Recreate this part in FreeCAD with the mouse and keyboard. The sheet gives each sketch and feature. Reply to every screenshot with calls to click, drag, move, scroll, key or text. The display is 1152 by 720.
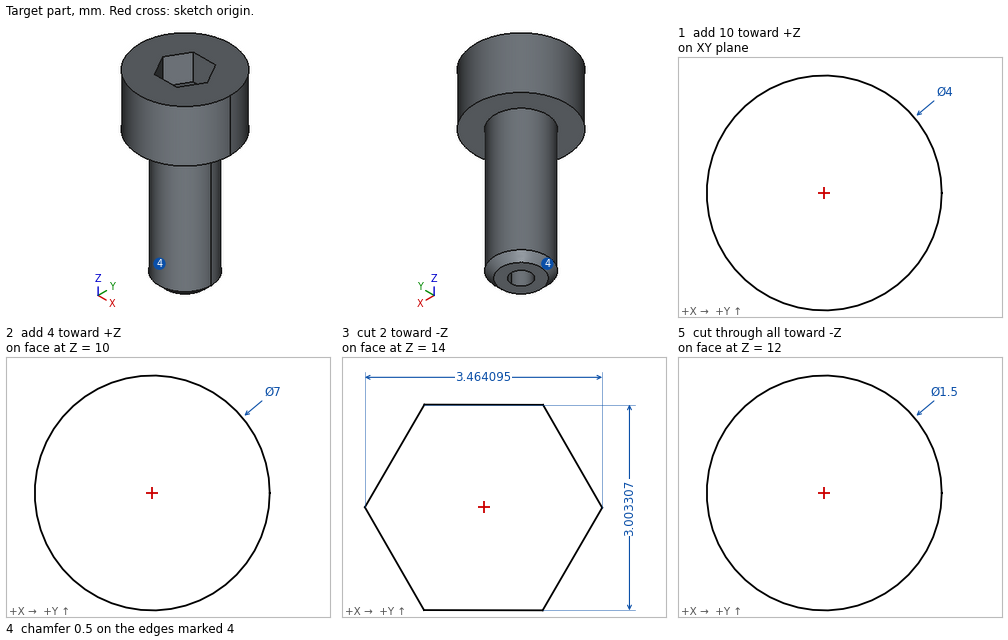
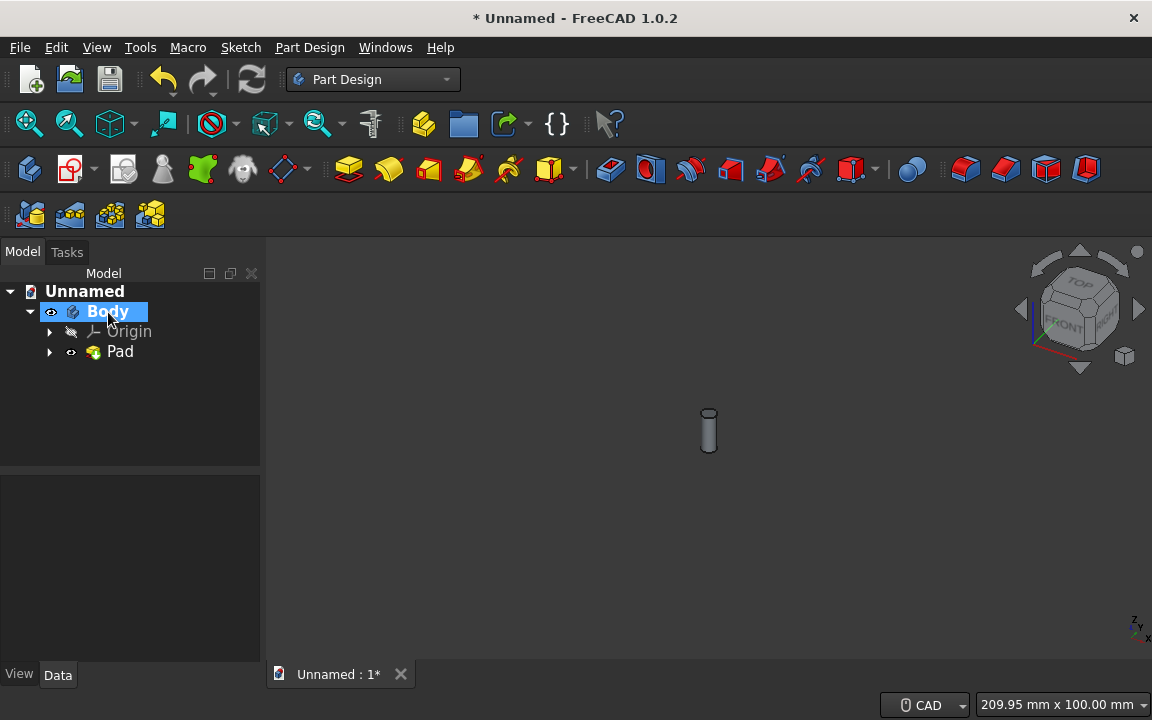
click(30, 124)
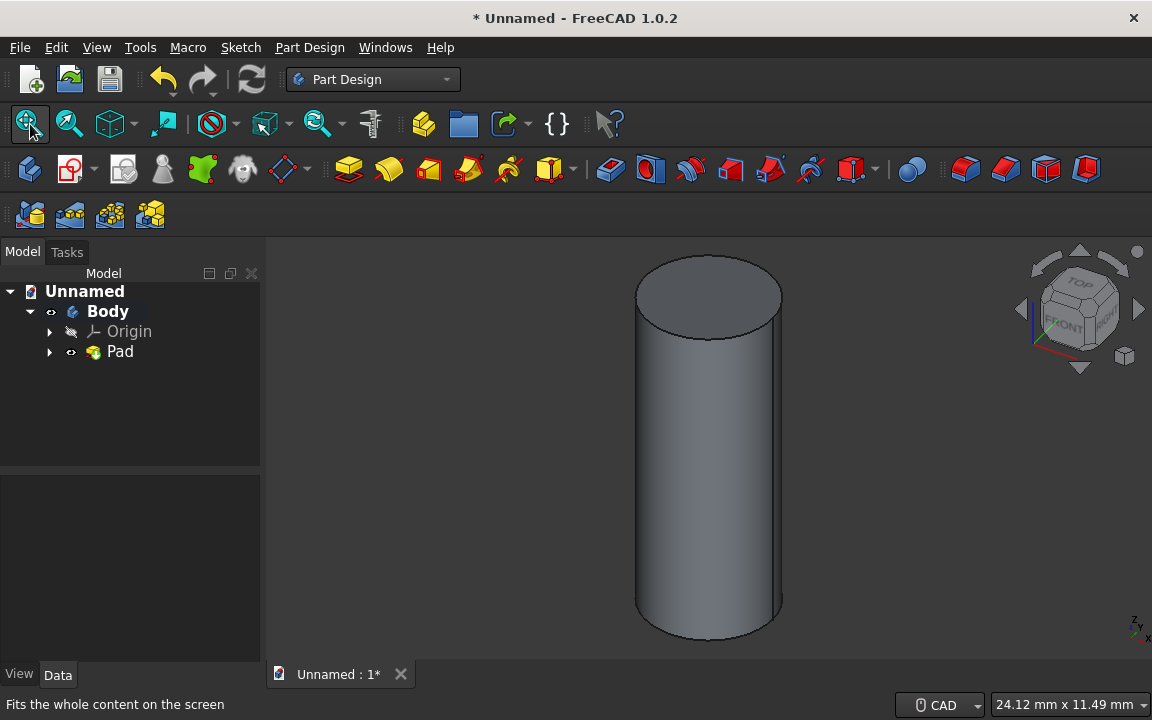
click(709, 296)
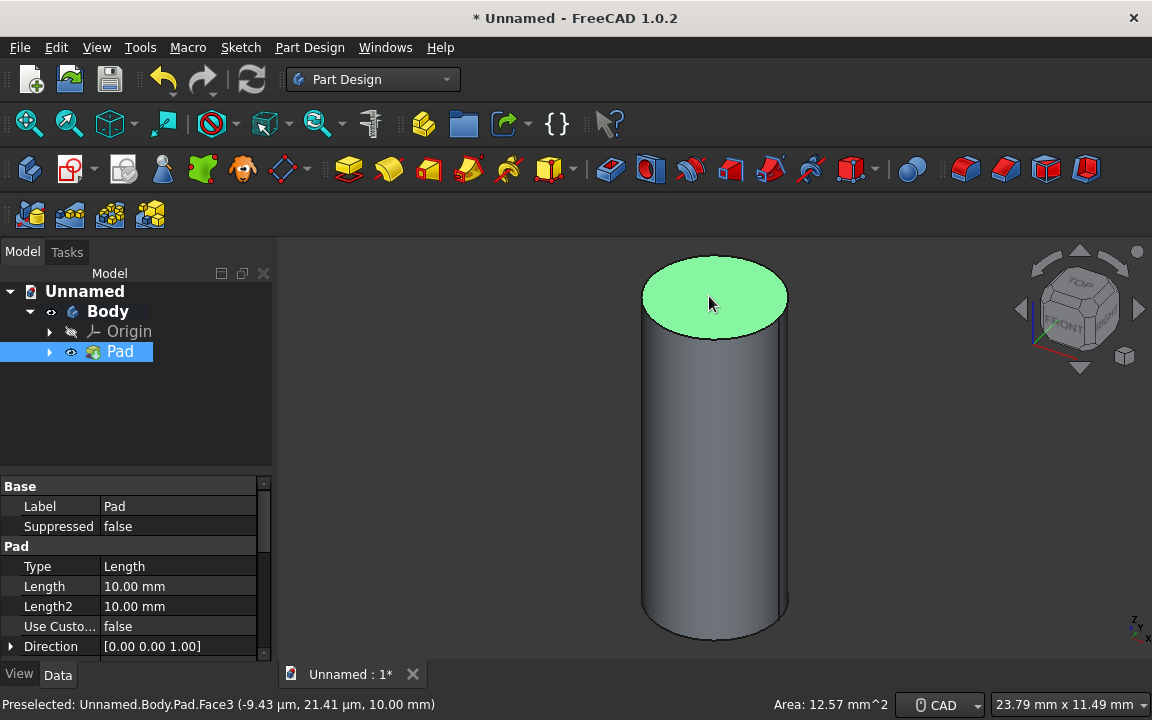
click(70, 170)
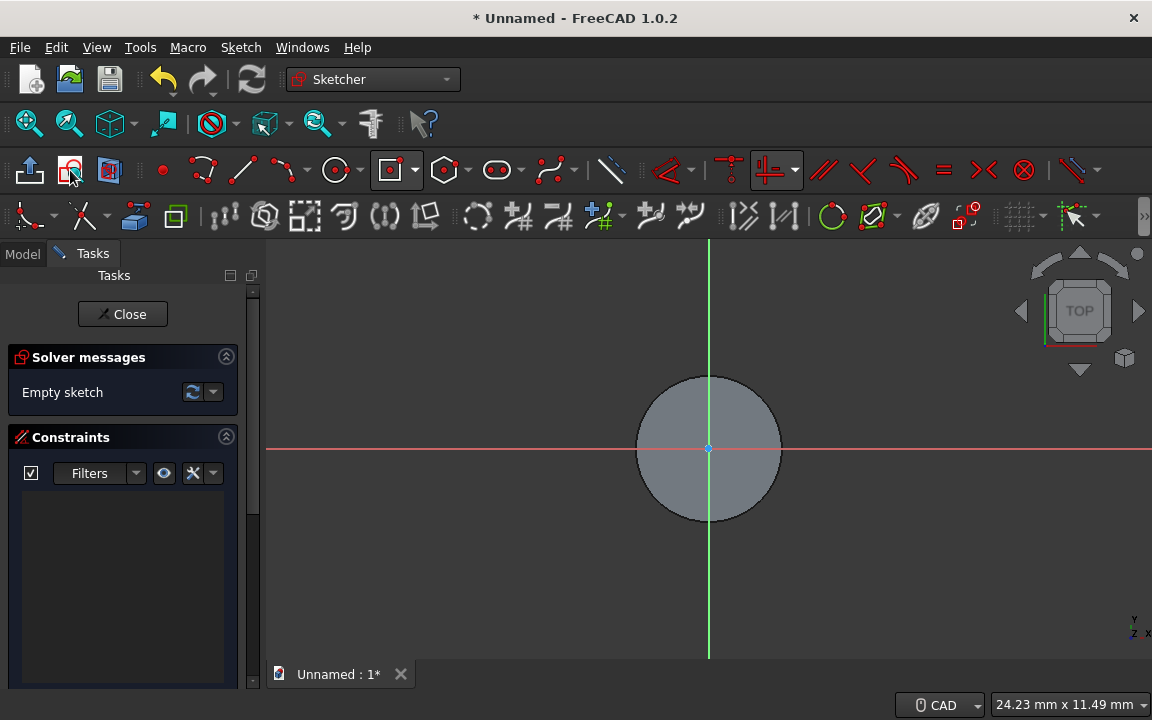
click(336, 170)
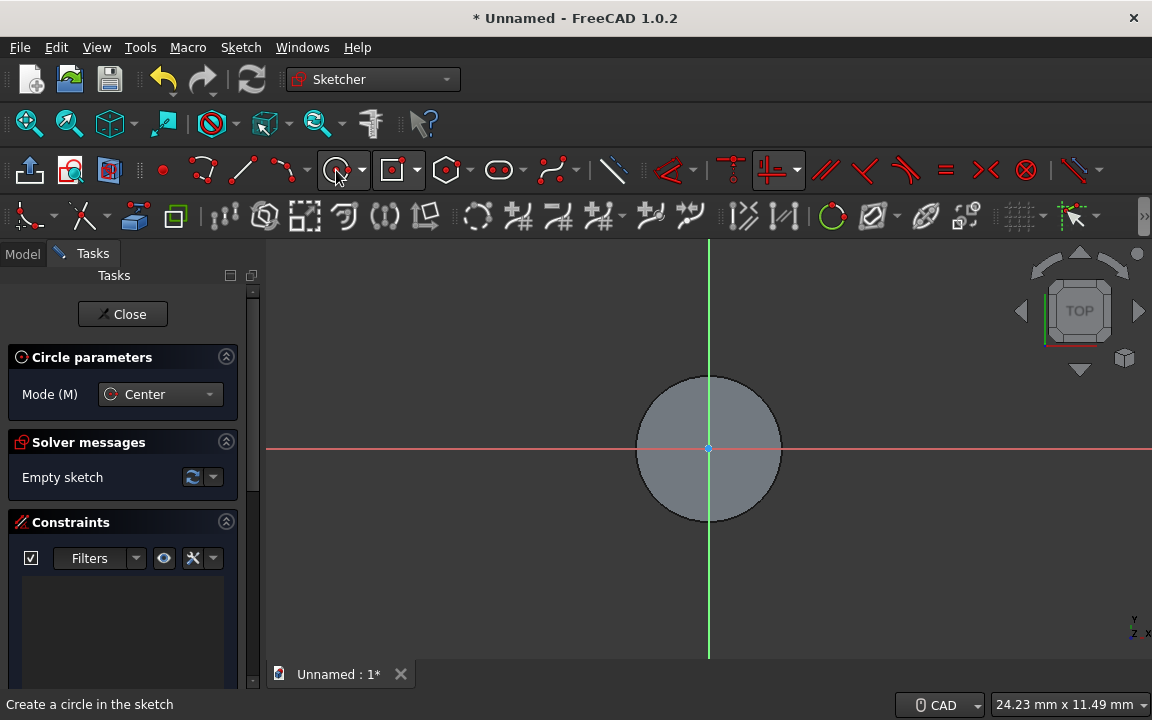
click(709, 449)
move(799, 359)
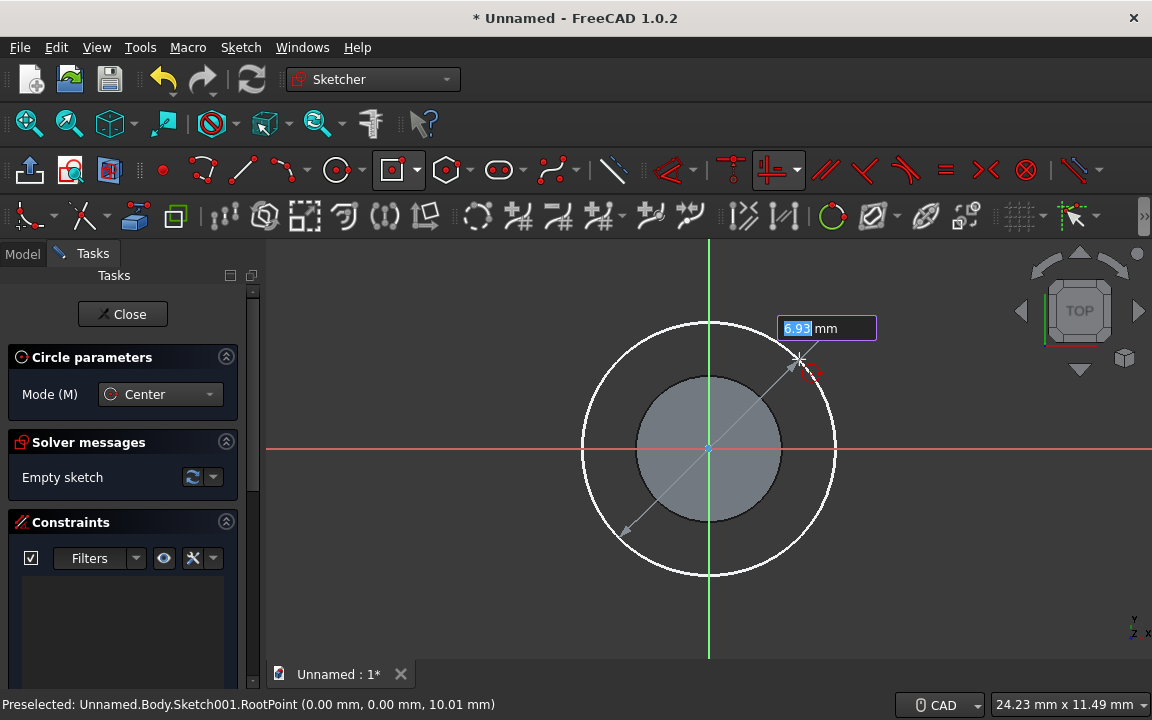
text(7)
key(Return)
key(Escape)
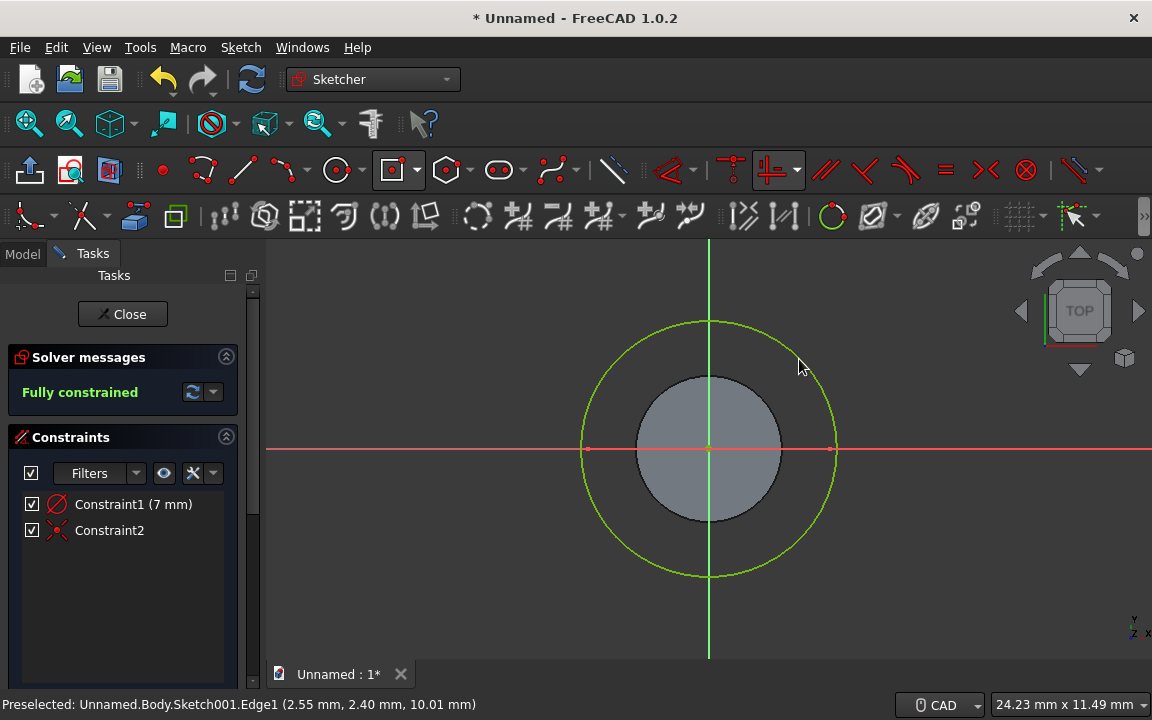
click(123, 314)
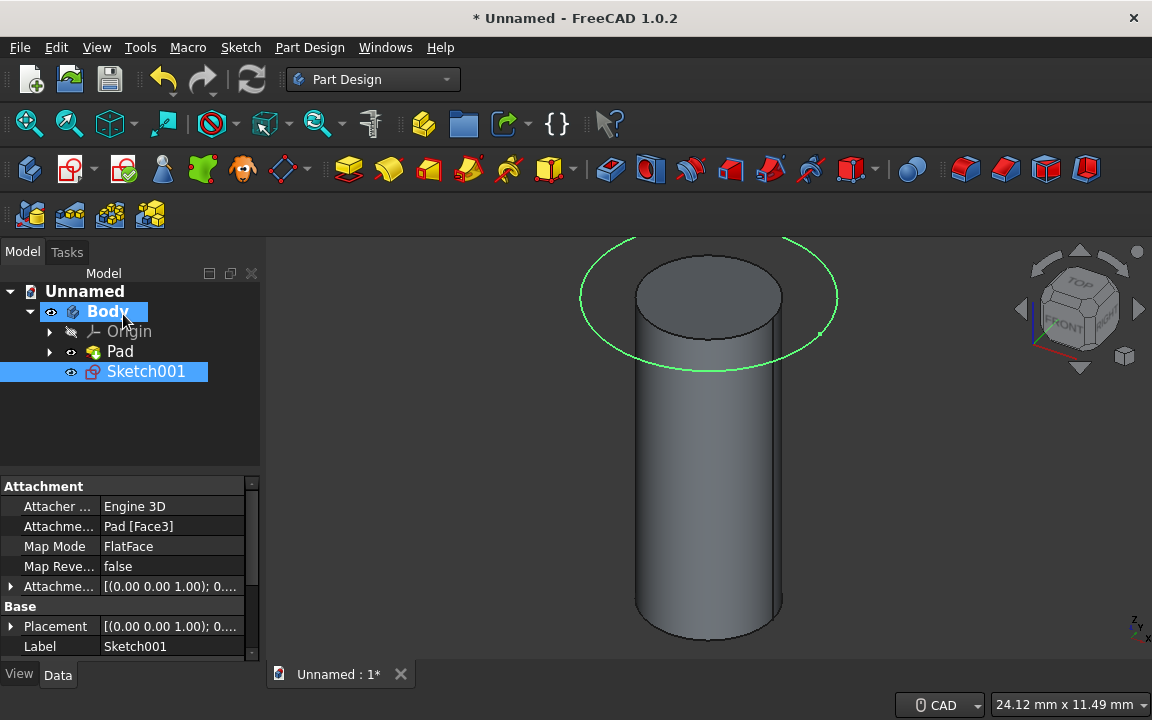
click(350, 170)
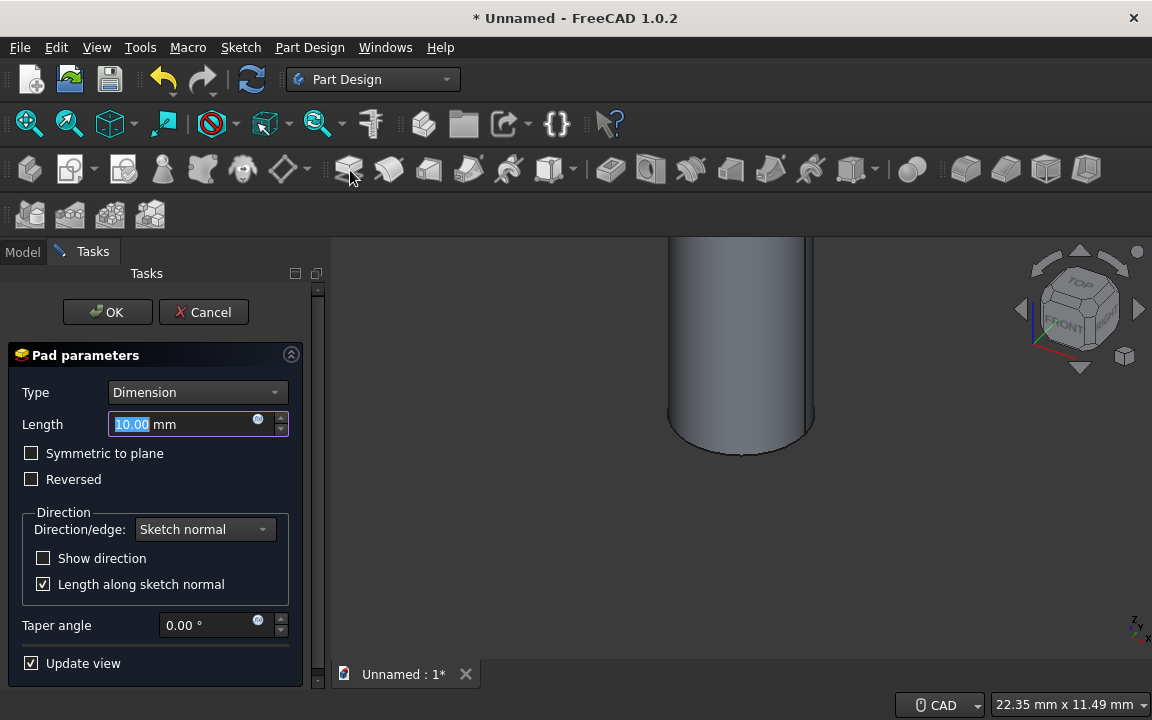
text(4)
key(Tab)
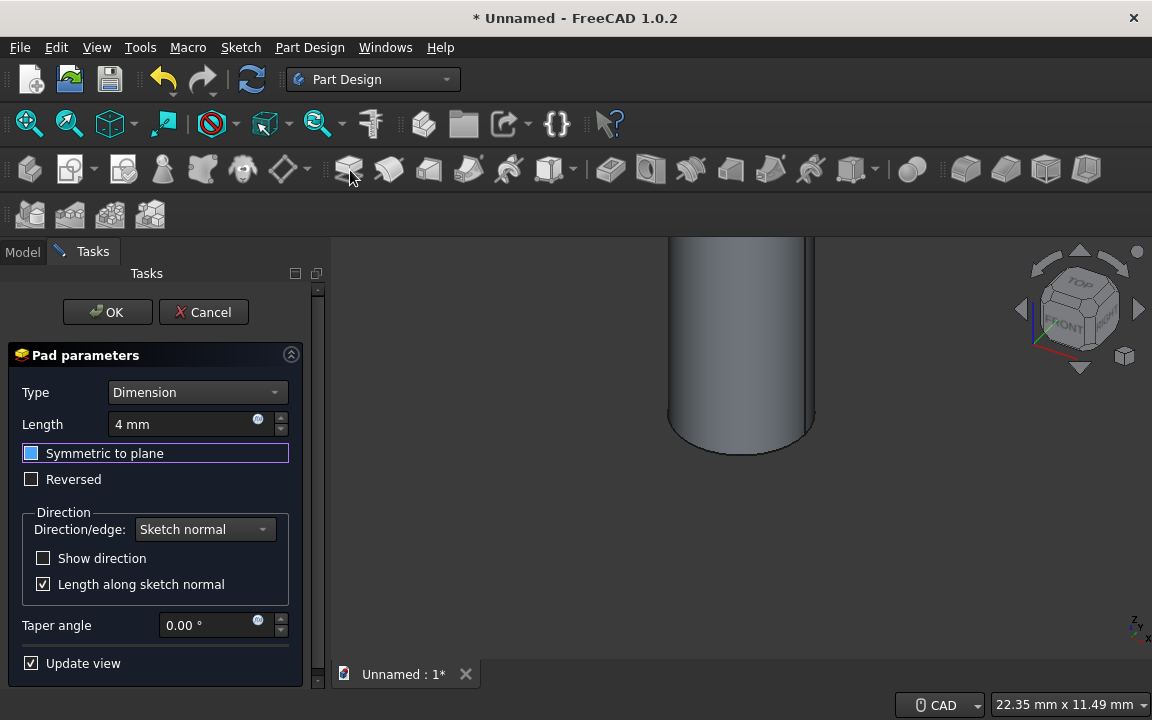
click(108, 312)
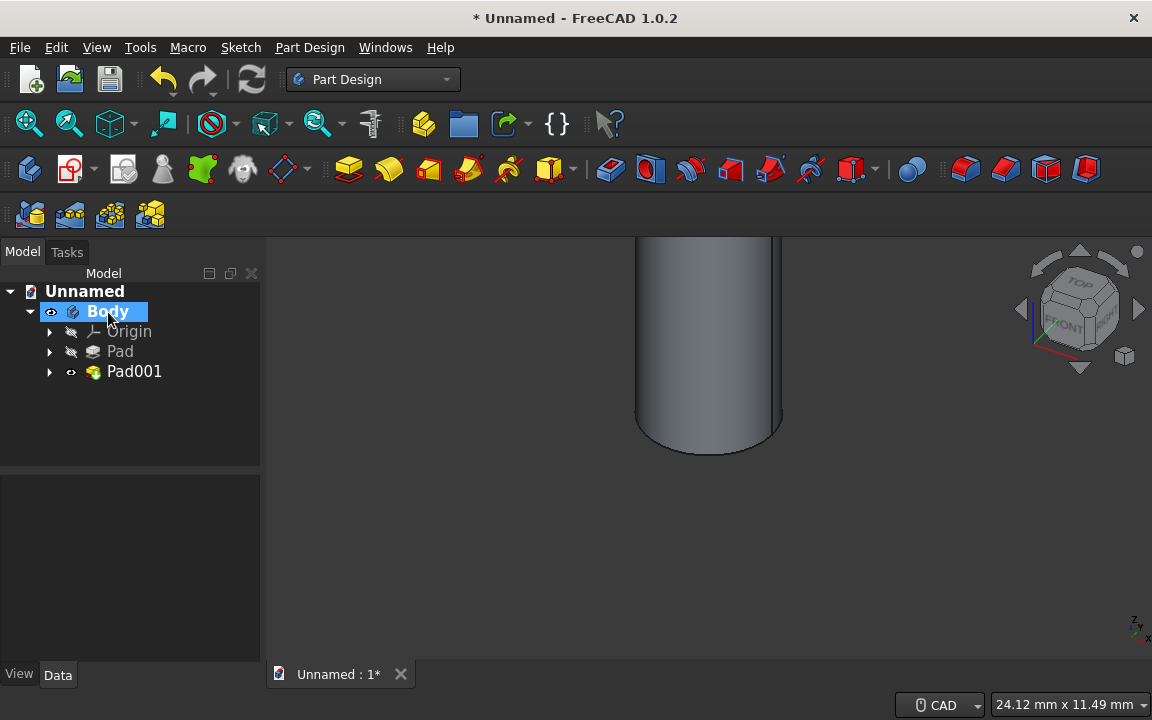
click(30, 124)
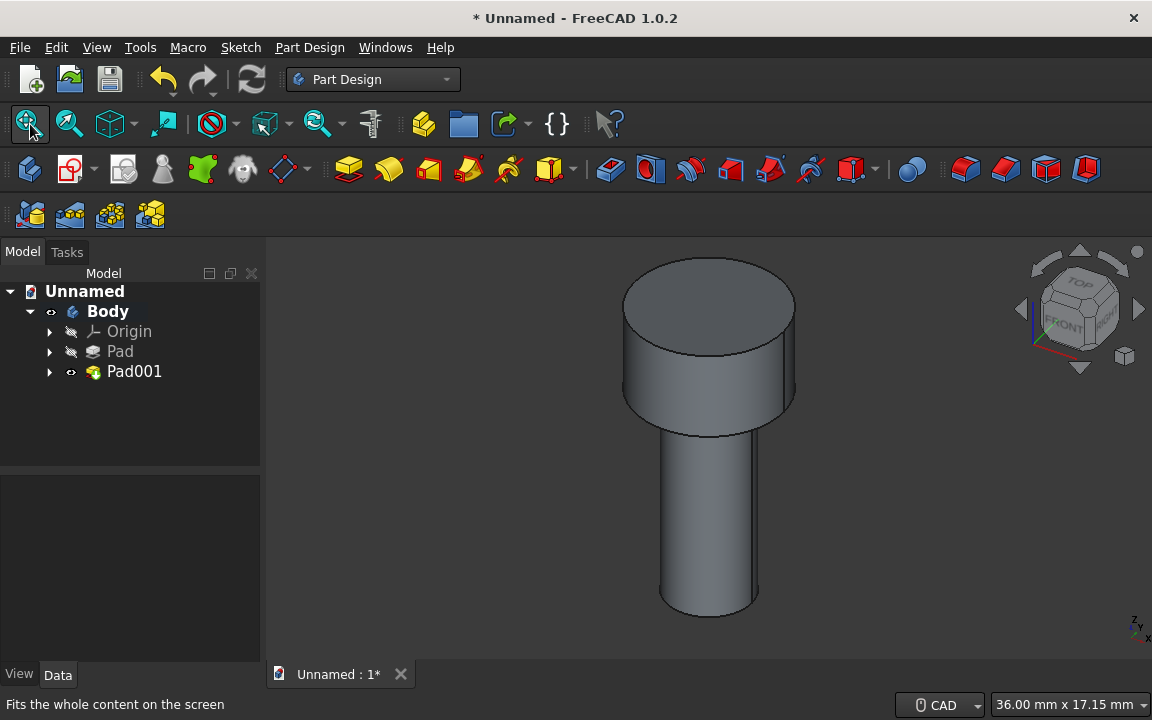
click(709, 306)